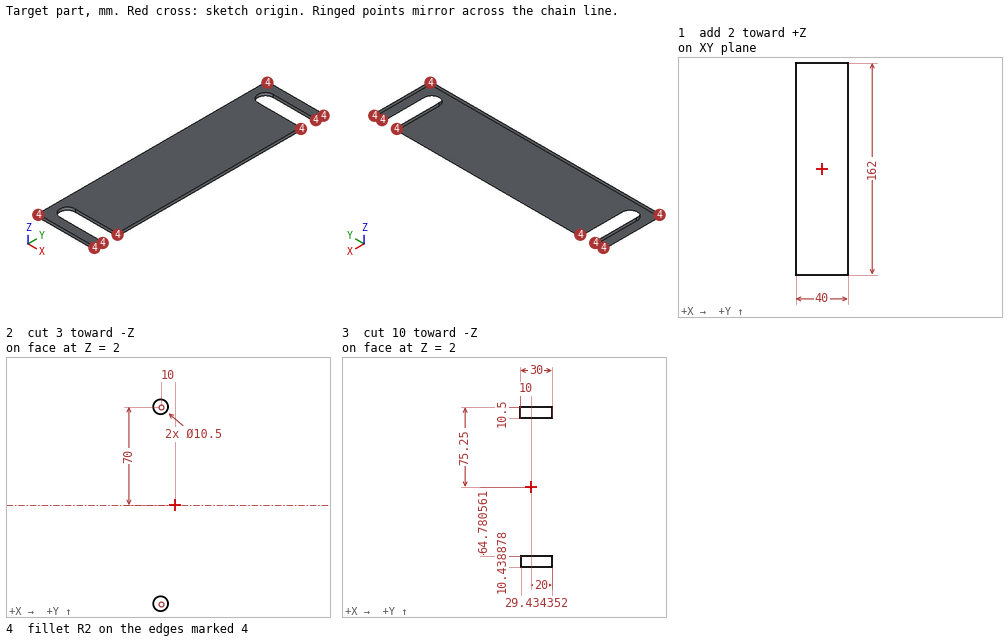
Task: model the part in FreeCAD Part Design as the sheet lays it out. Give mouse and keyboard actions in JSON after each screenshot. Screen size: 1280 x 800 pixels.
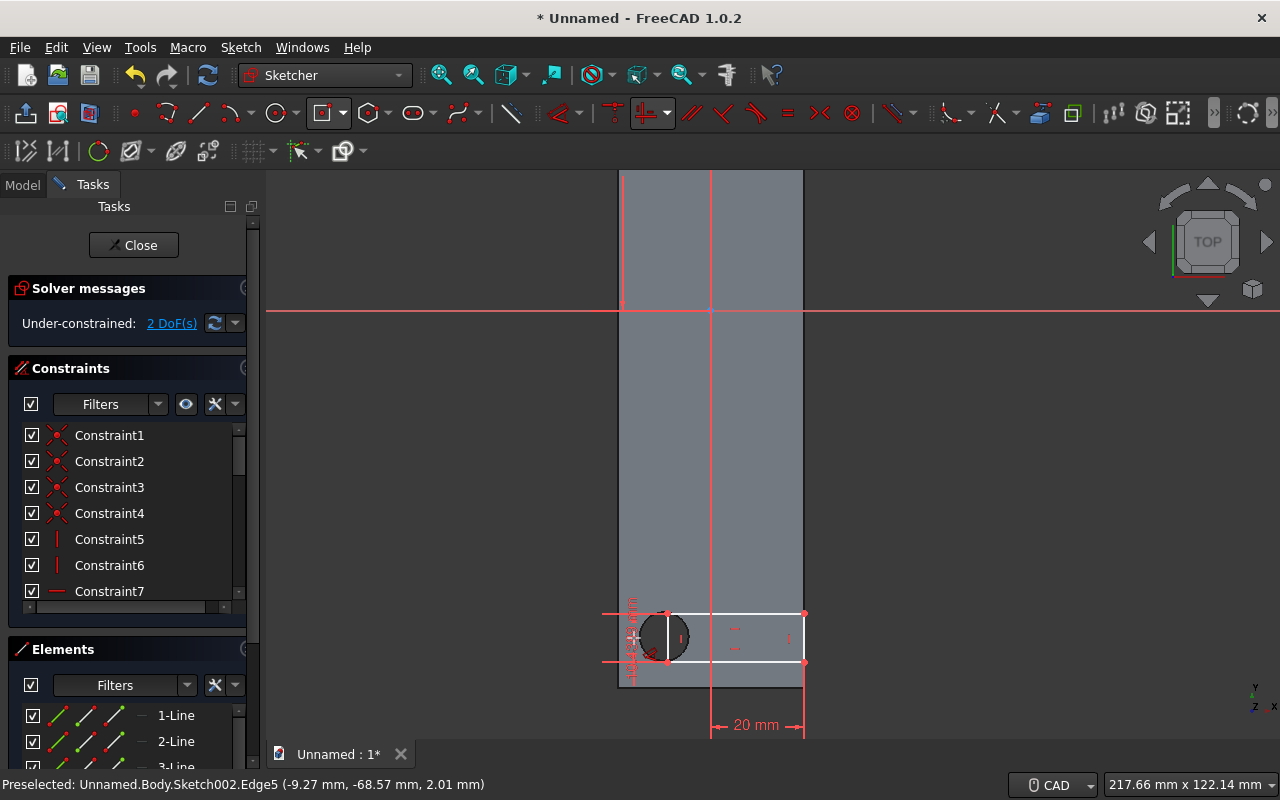
{"action": "left_click", "coordinate": [709, 662]}
{"action": "left_click", "coordinate": [736, 696]}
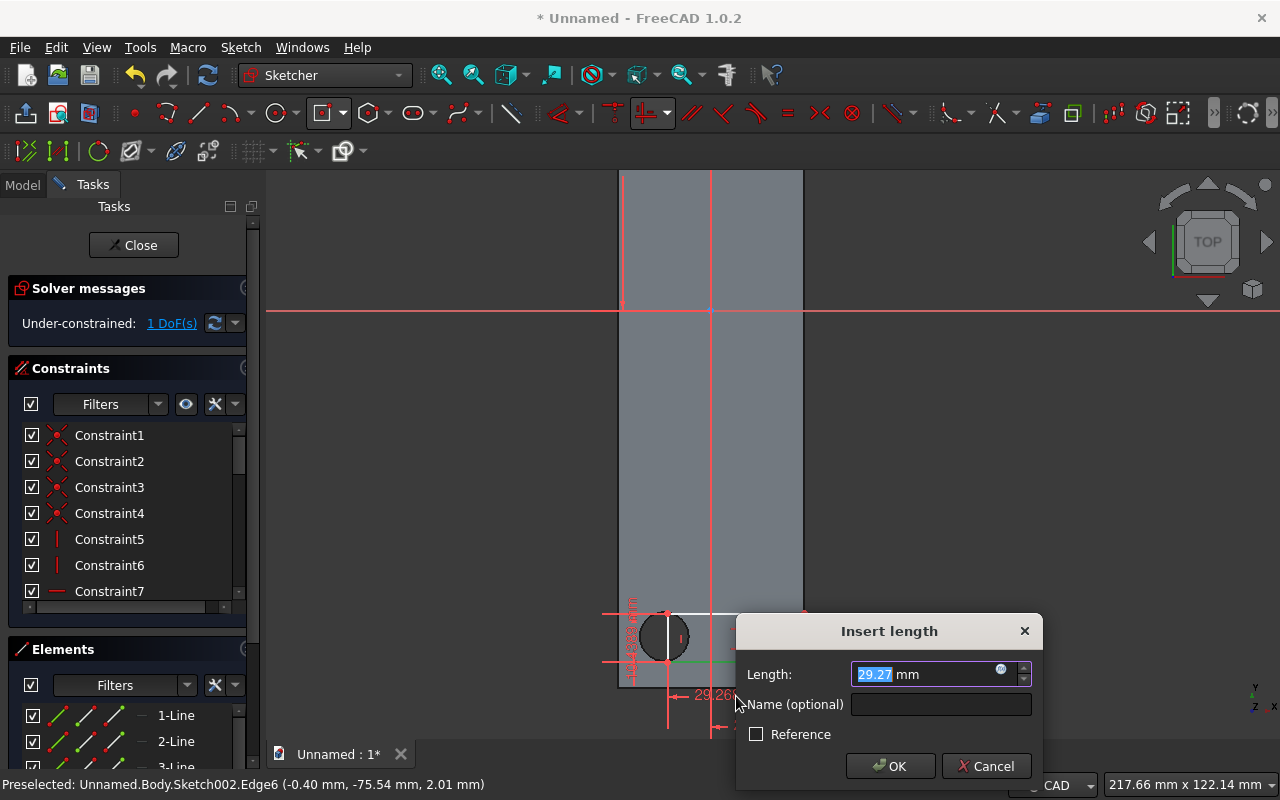
{"action": "type", "text": "29.434352"}
{"action": "key", "text": "Return"}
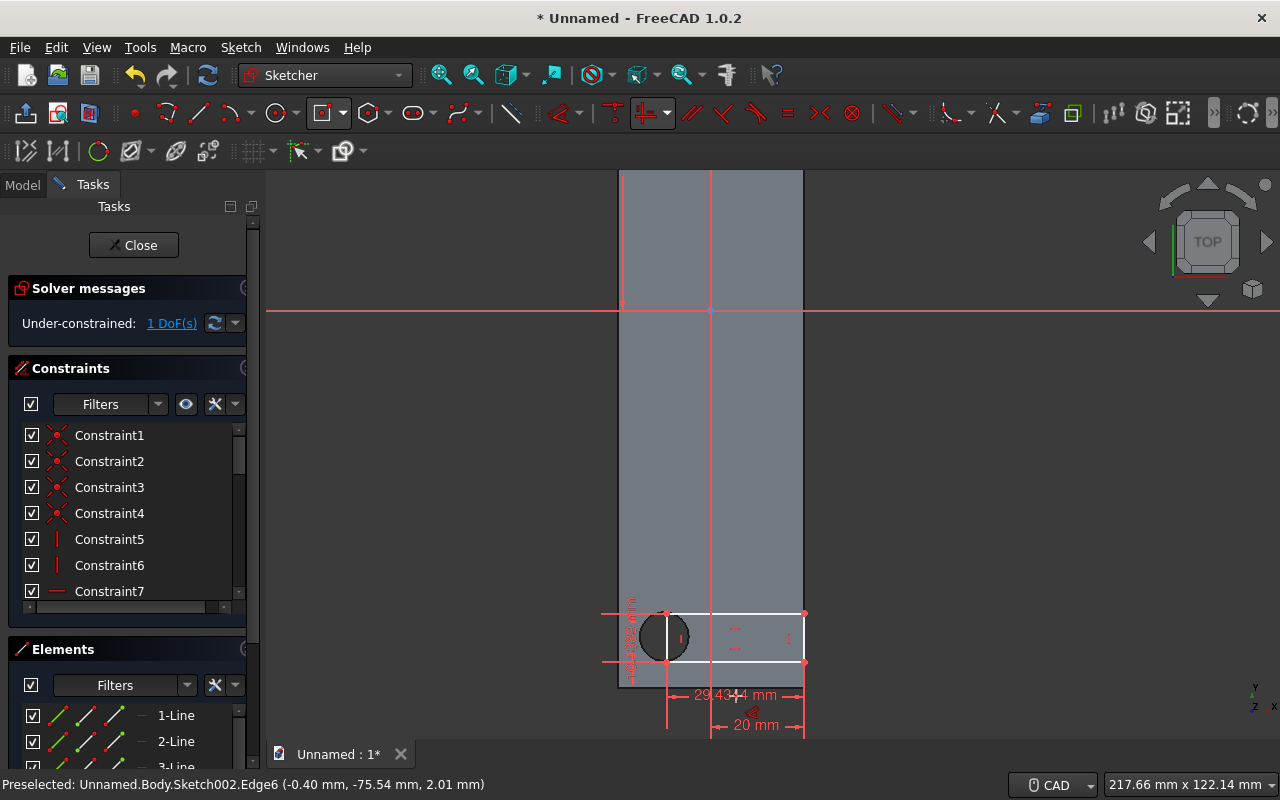
{"action": "left_click", "coordinate": [667, 614]}
{"action": "left_click", "coordinate": [633, 462]}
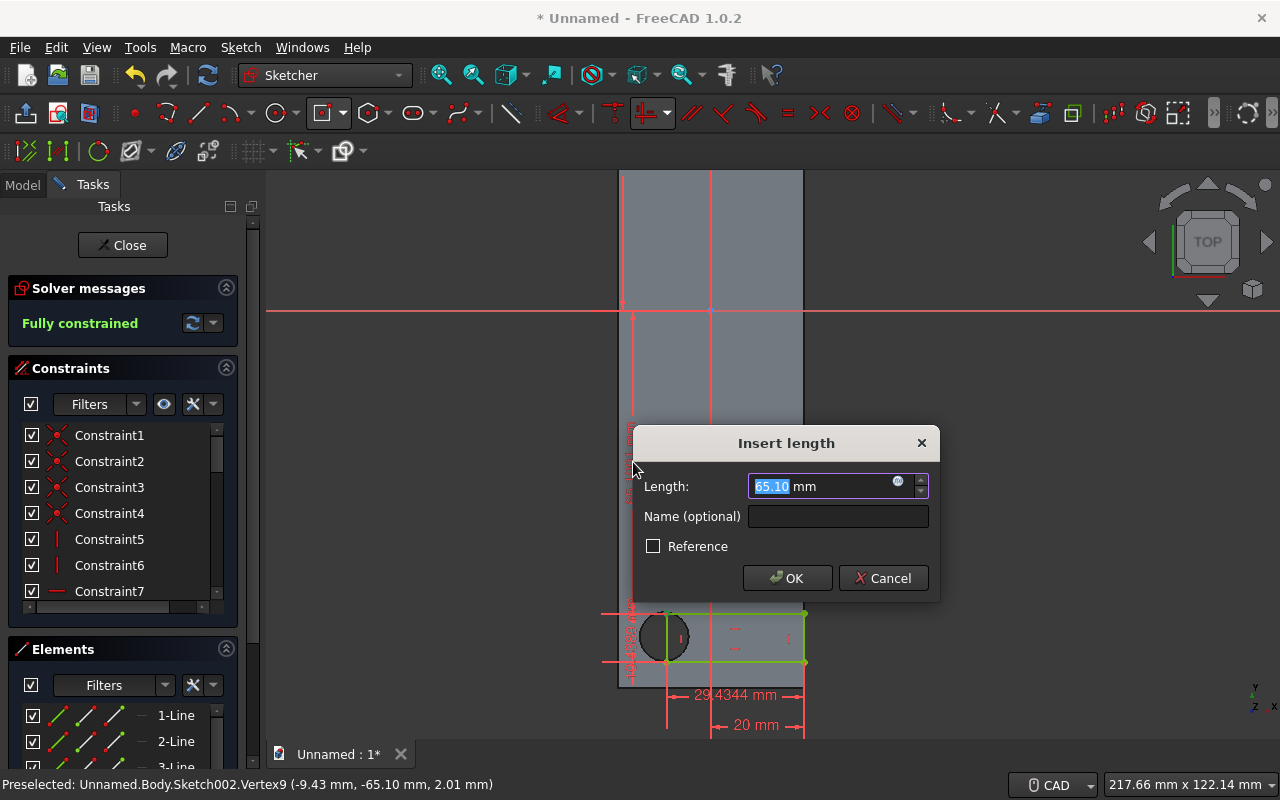
{"action": "type", "text": "64.780561"}
{"action": "key", "text": "Return"}
{"action": "key", "text": "Escape"}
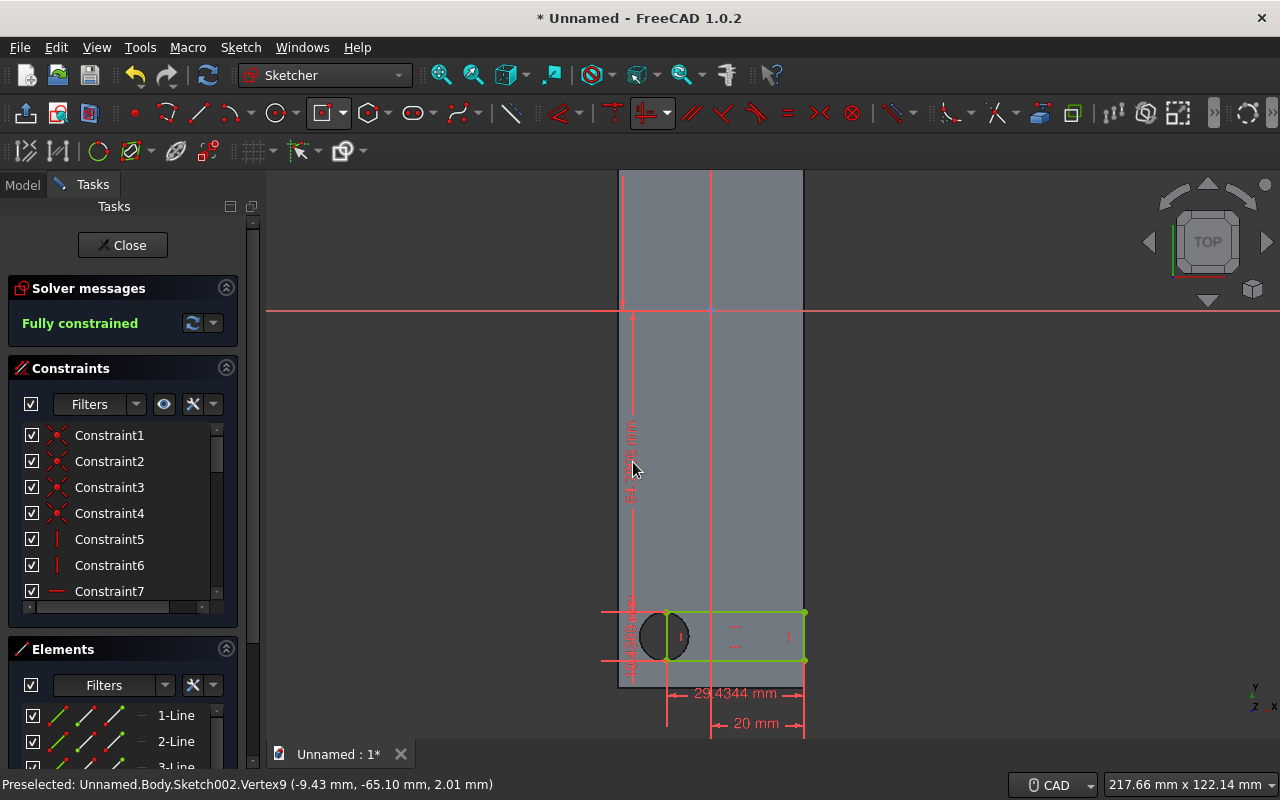
{"action": "left_click", "coordinate": [123, 245]}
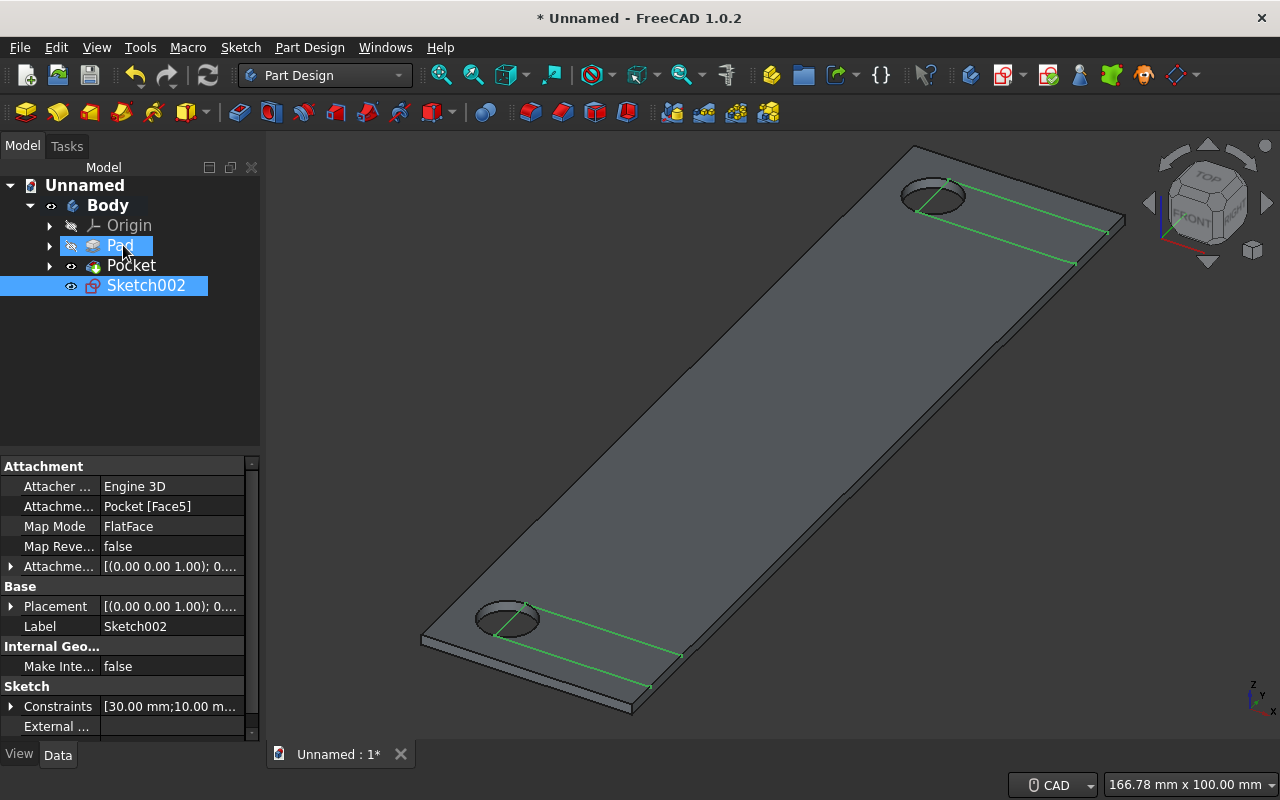
{"action": "left_click", "coordinate": [240, 112]}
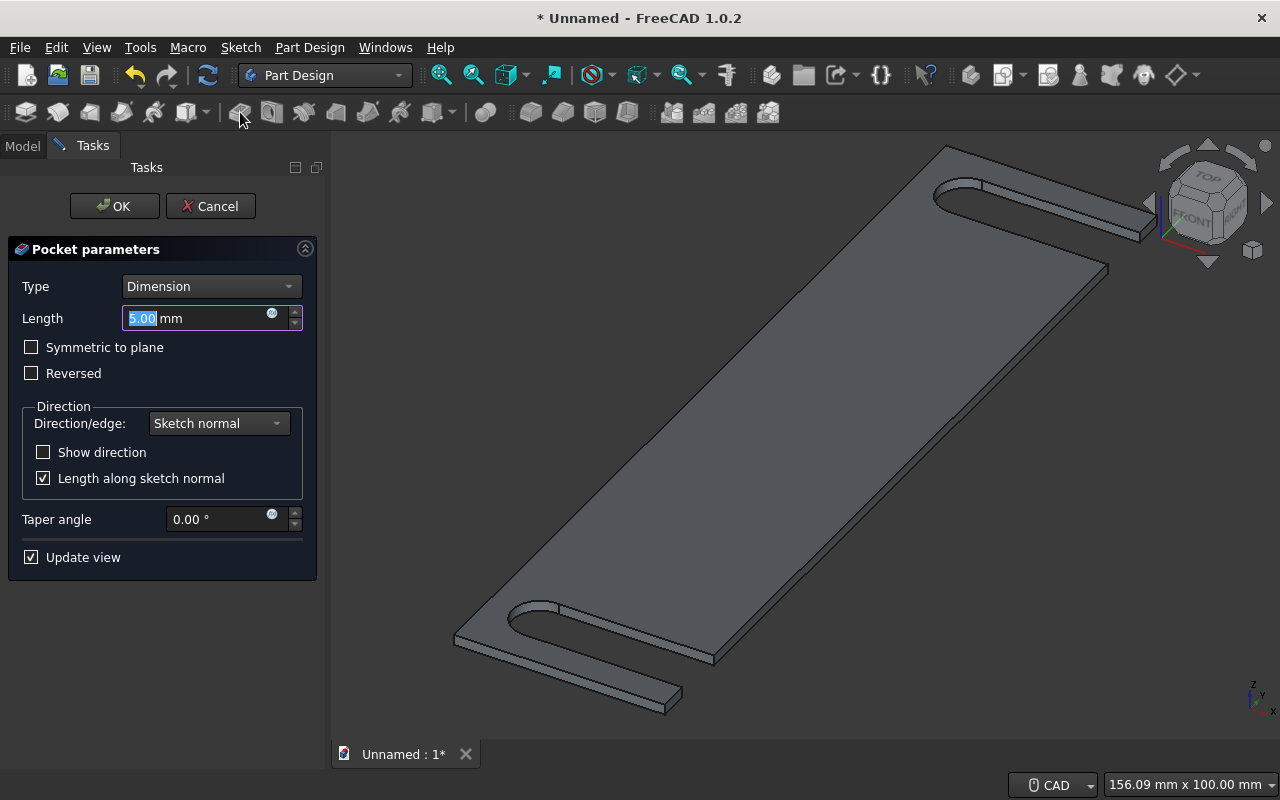
{"action": "type", "text": "10"}
{"action": "key", "text": "Tab"}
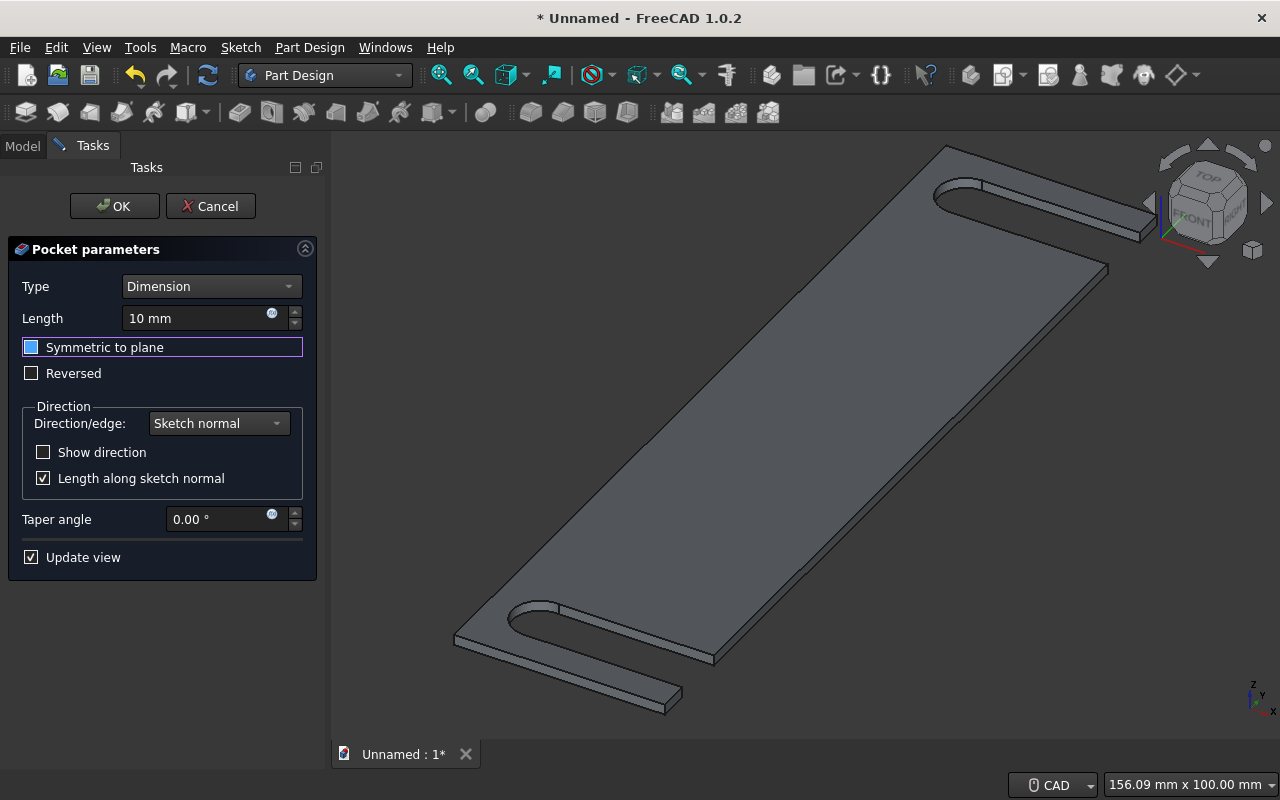
{"action": "left_click", "coordinate": [115, 206]}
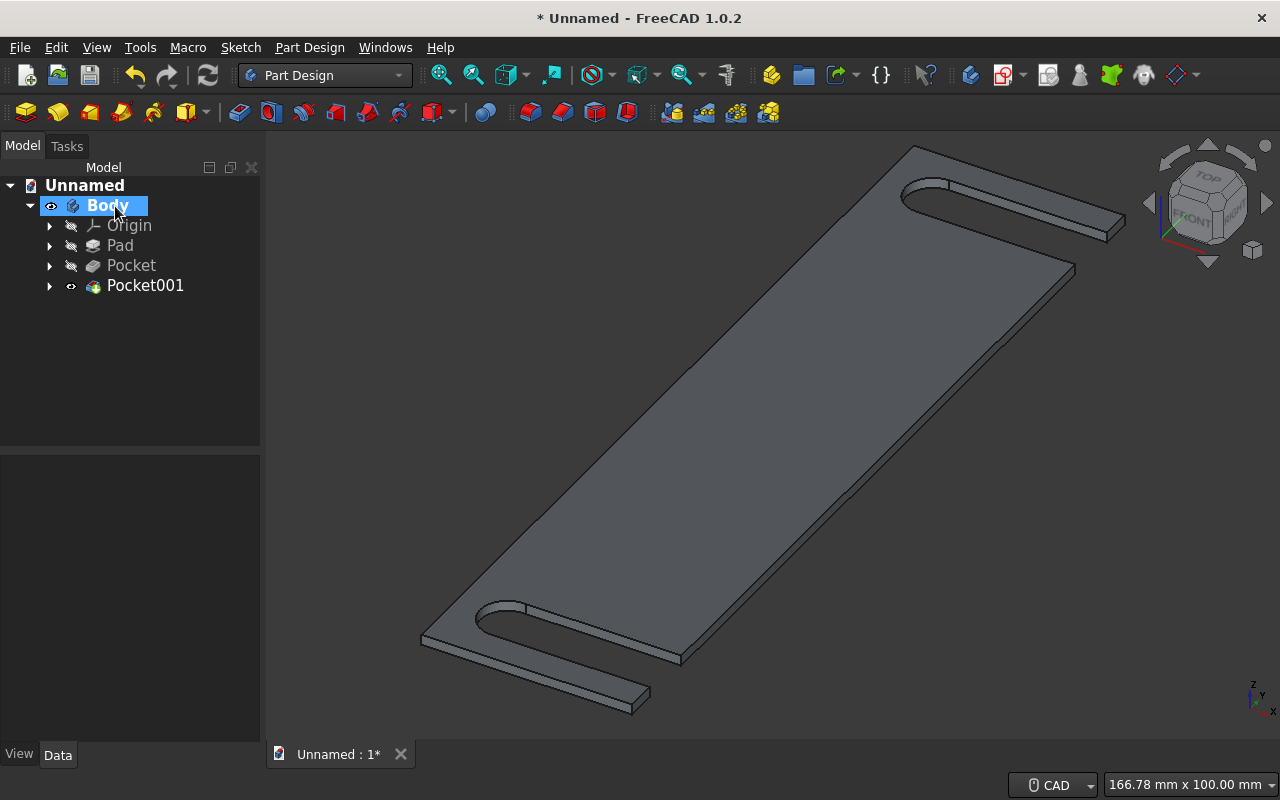
{"action": "left_click", "coordinate": [1107, 238]}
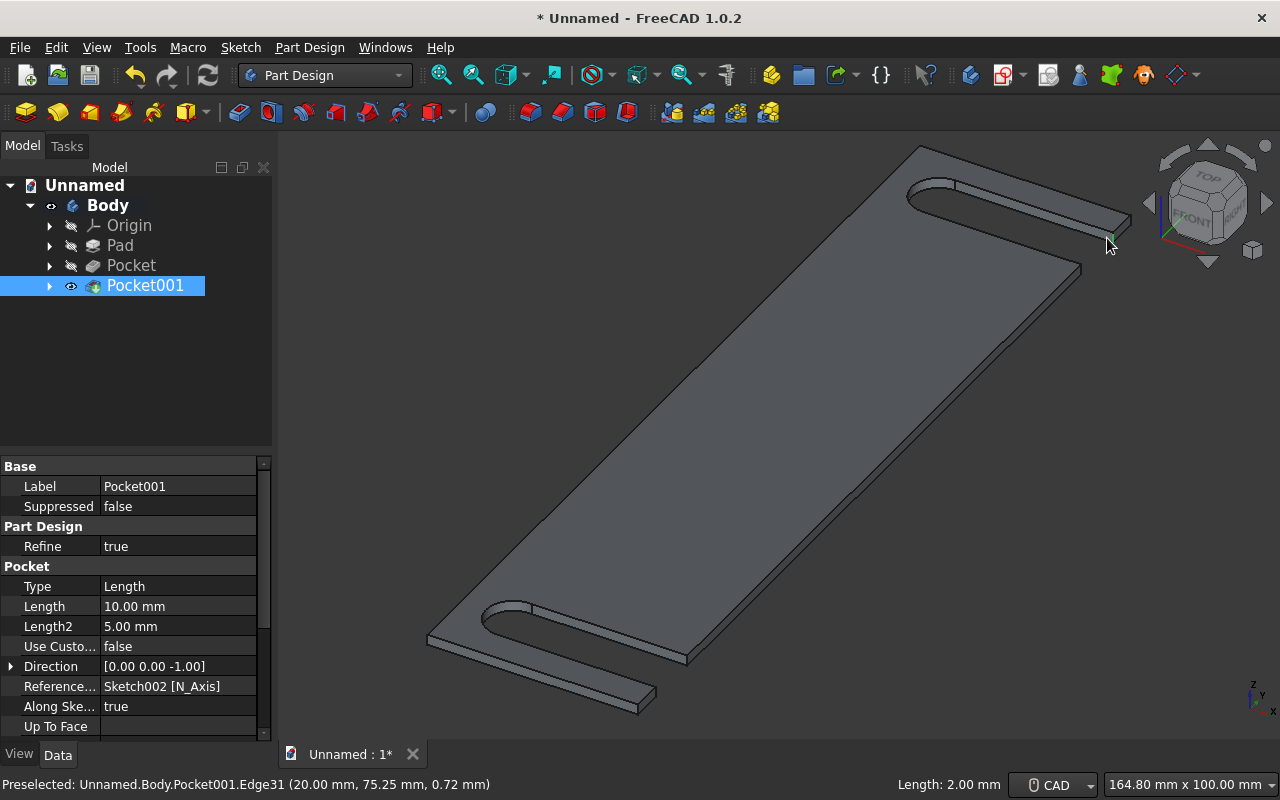
{"action": "left_click", "coordinate": [687, 661], "text": "ctrl"}